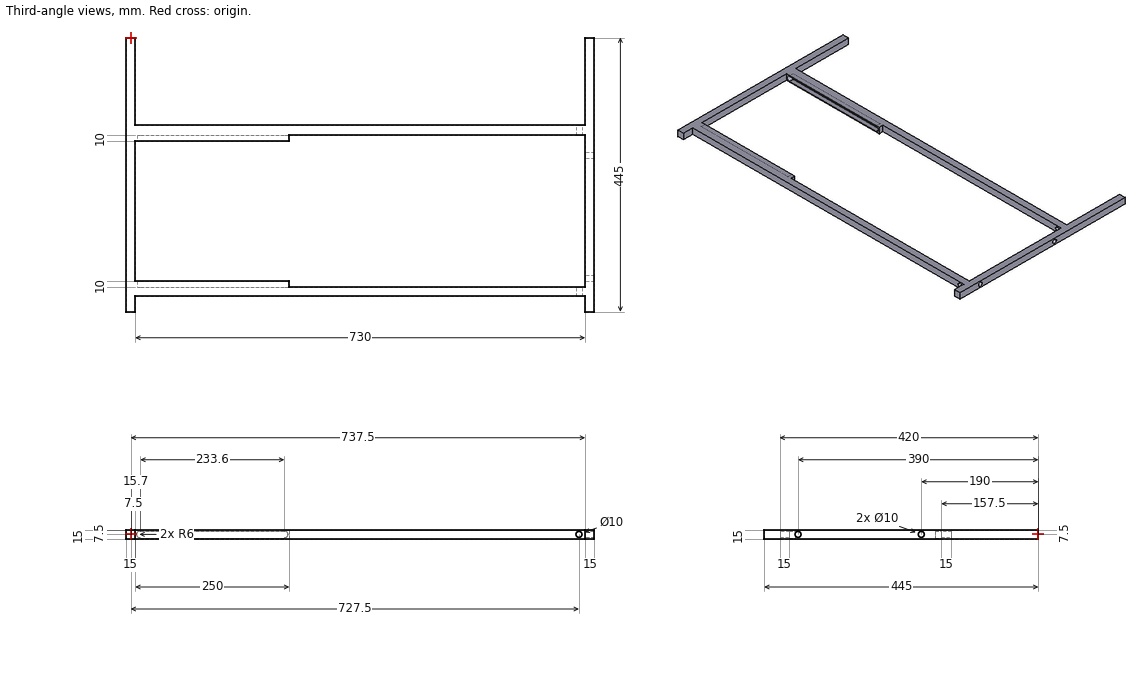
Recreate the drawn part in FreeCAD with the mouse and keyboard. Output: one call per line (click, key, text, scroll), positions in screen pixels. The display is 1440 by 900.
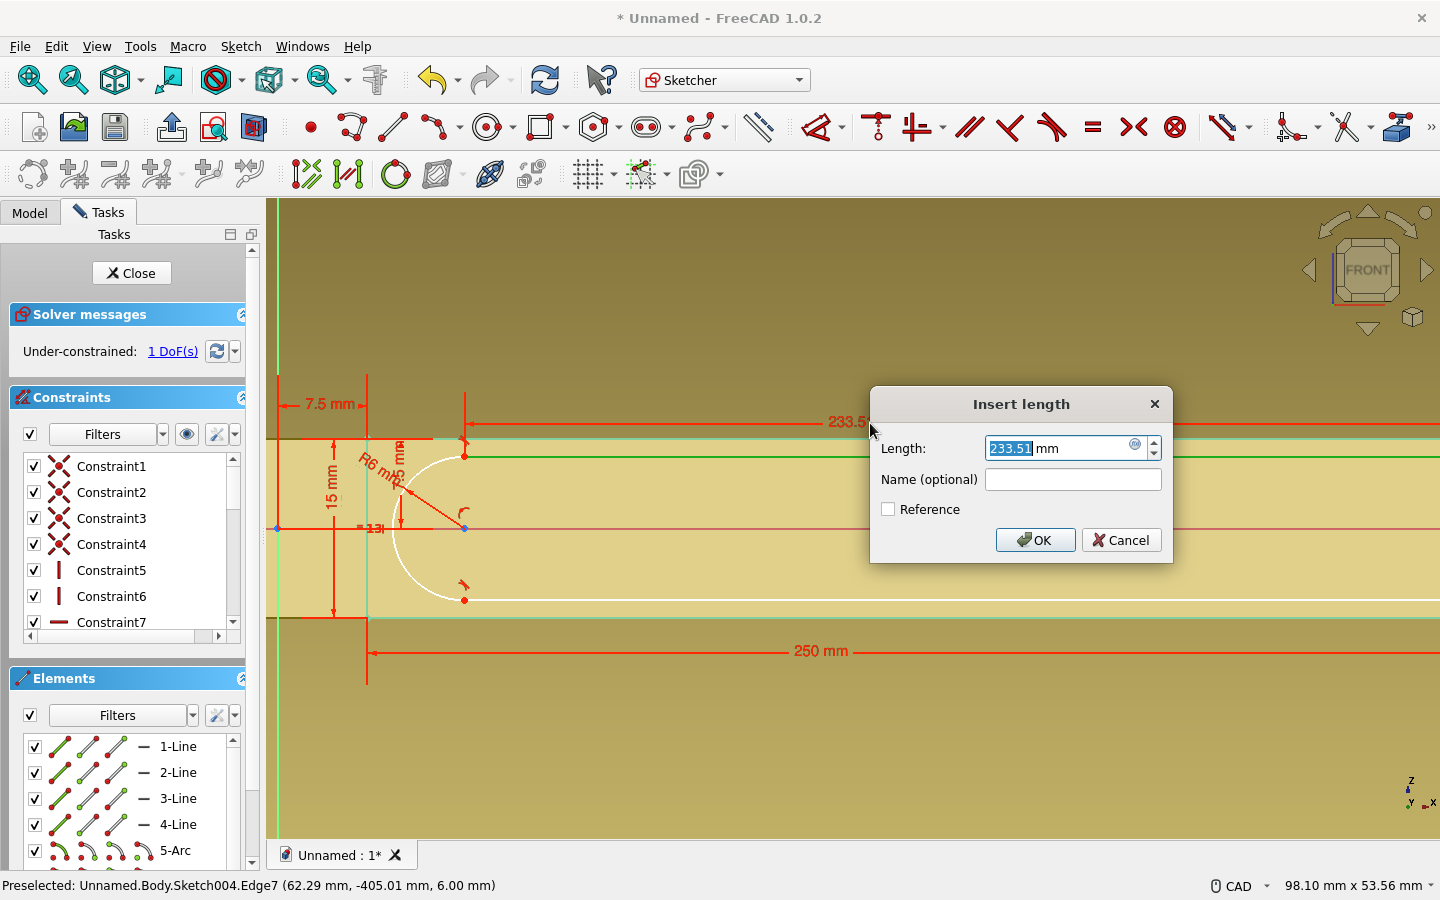
text(233.6)
key(Return)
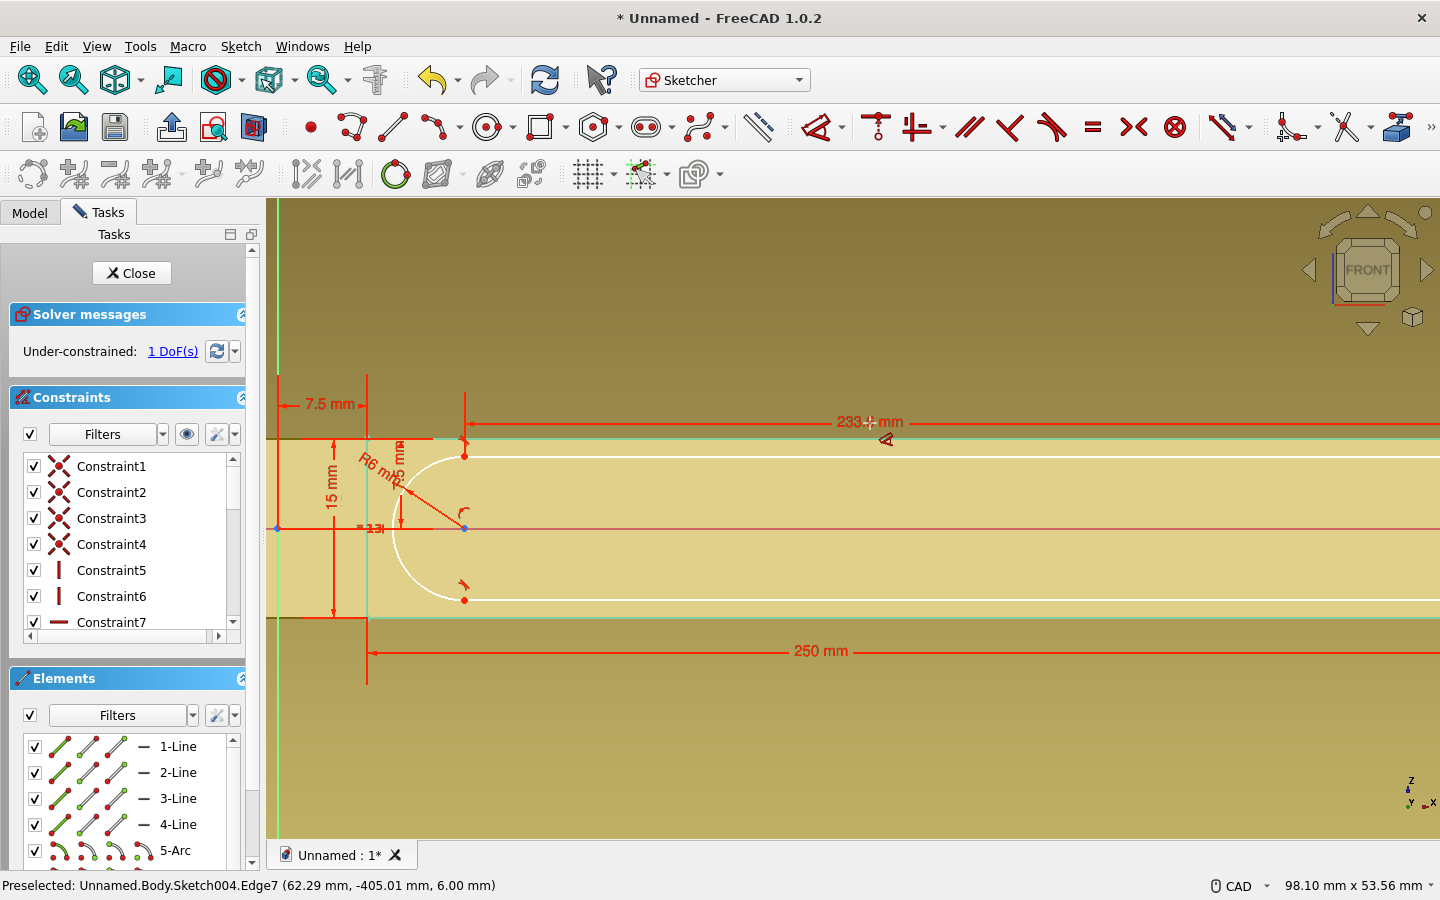
scroll(446, 515, down, 7)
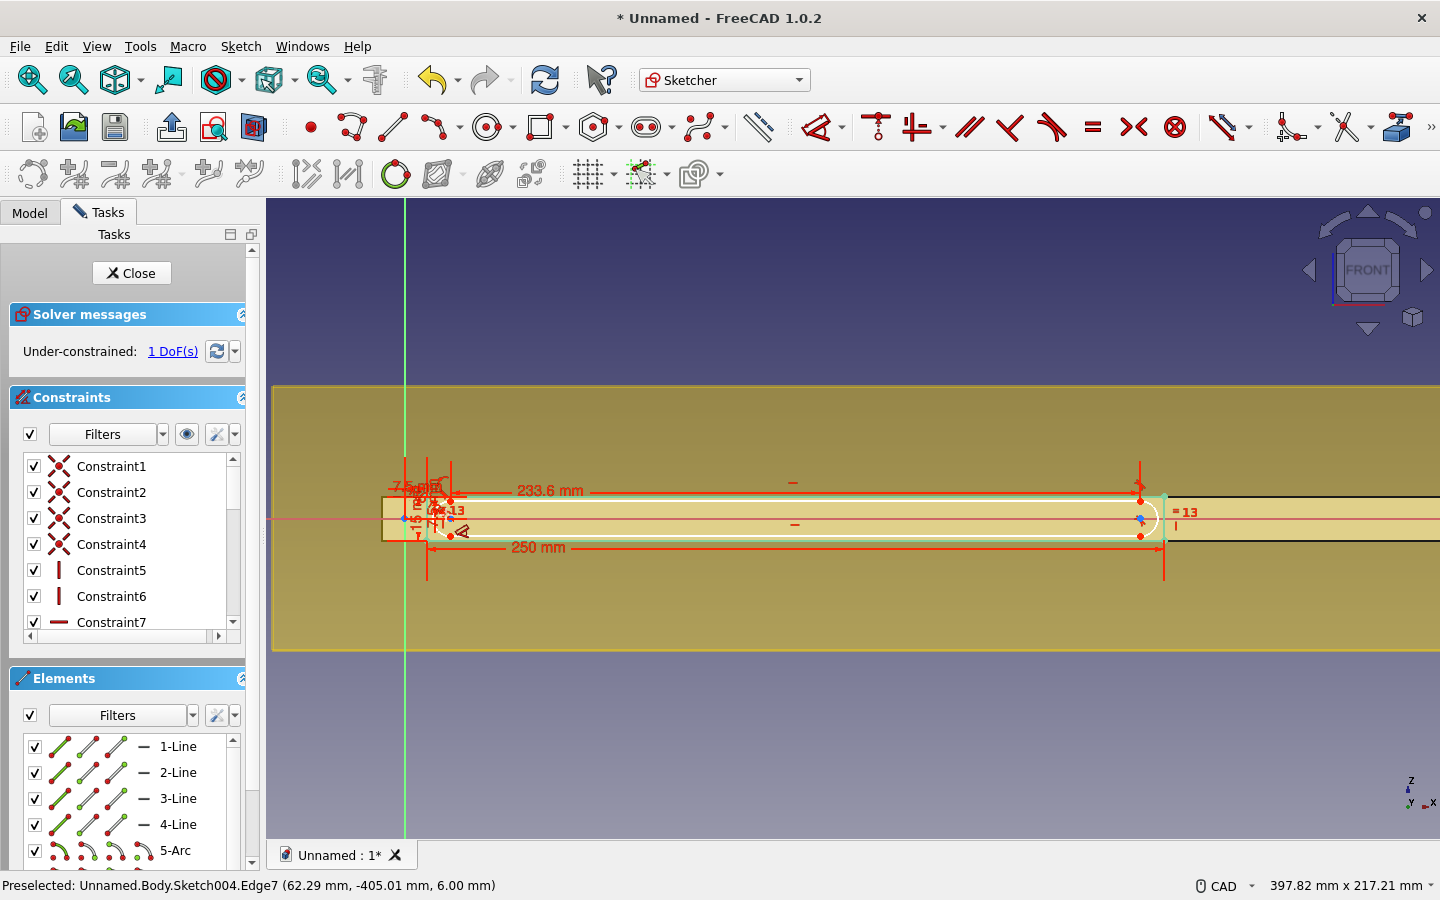
click(451, 501)
click(428, 467)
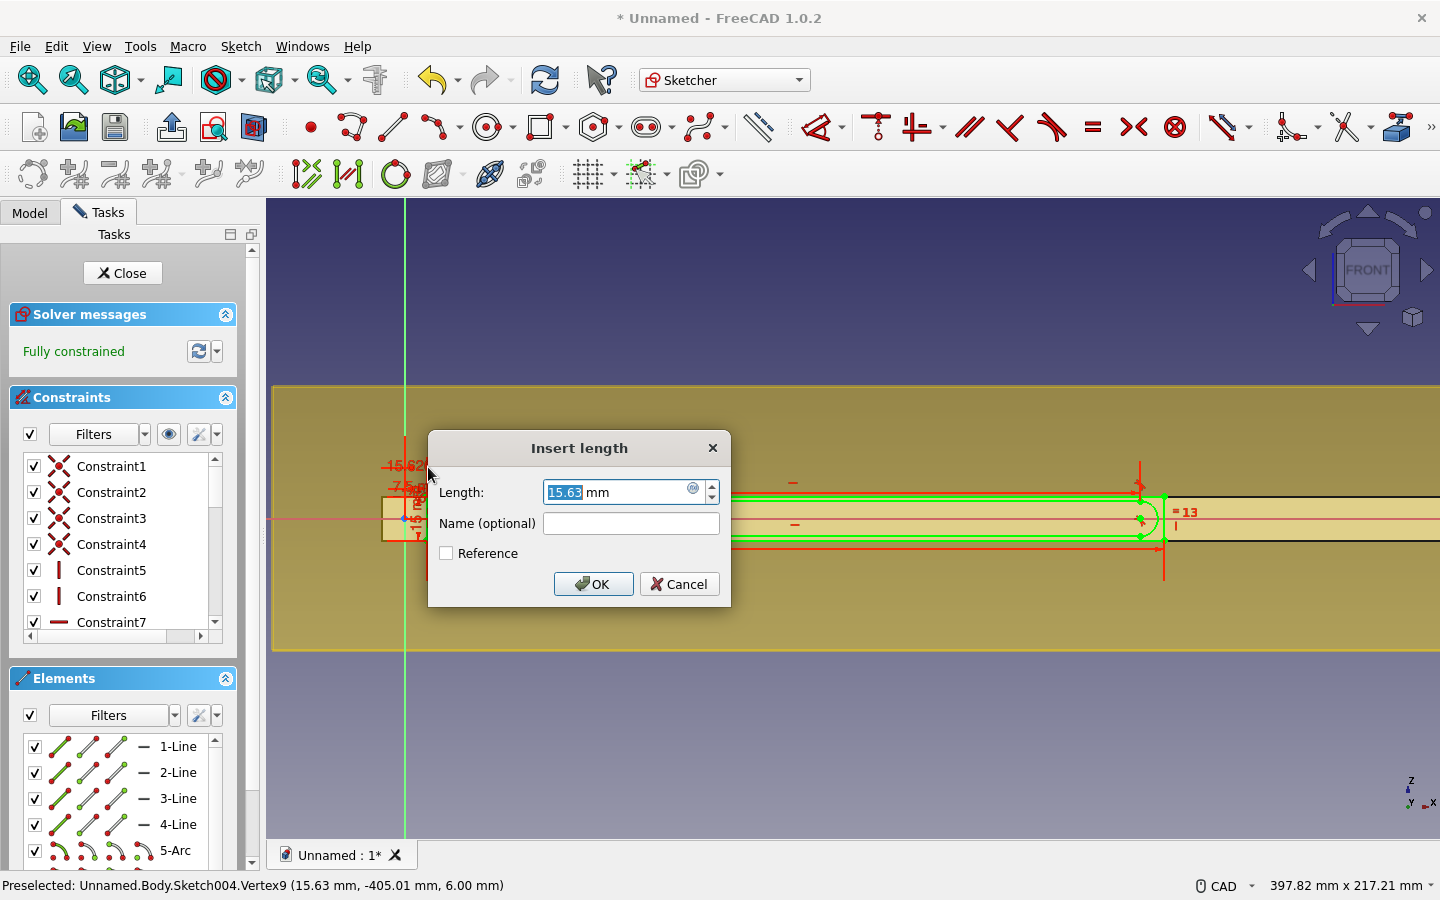
text(15.7)
key(Return)
key(Escape)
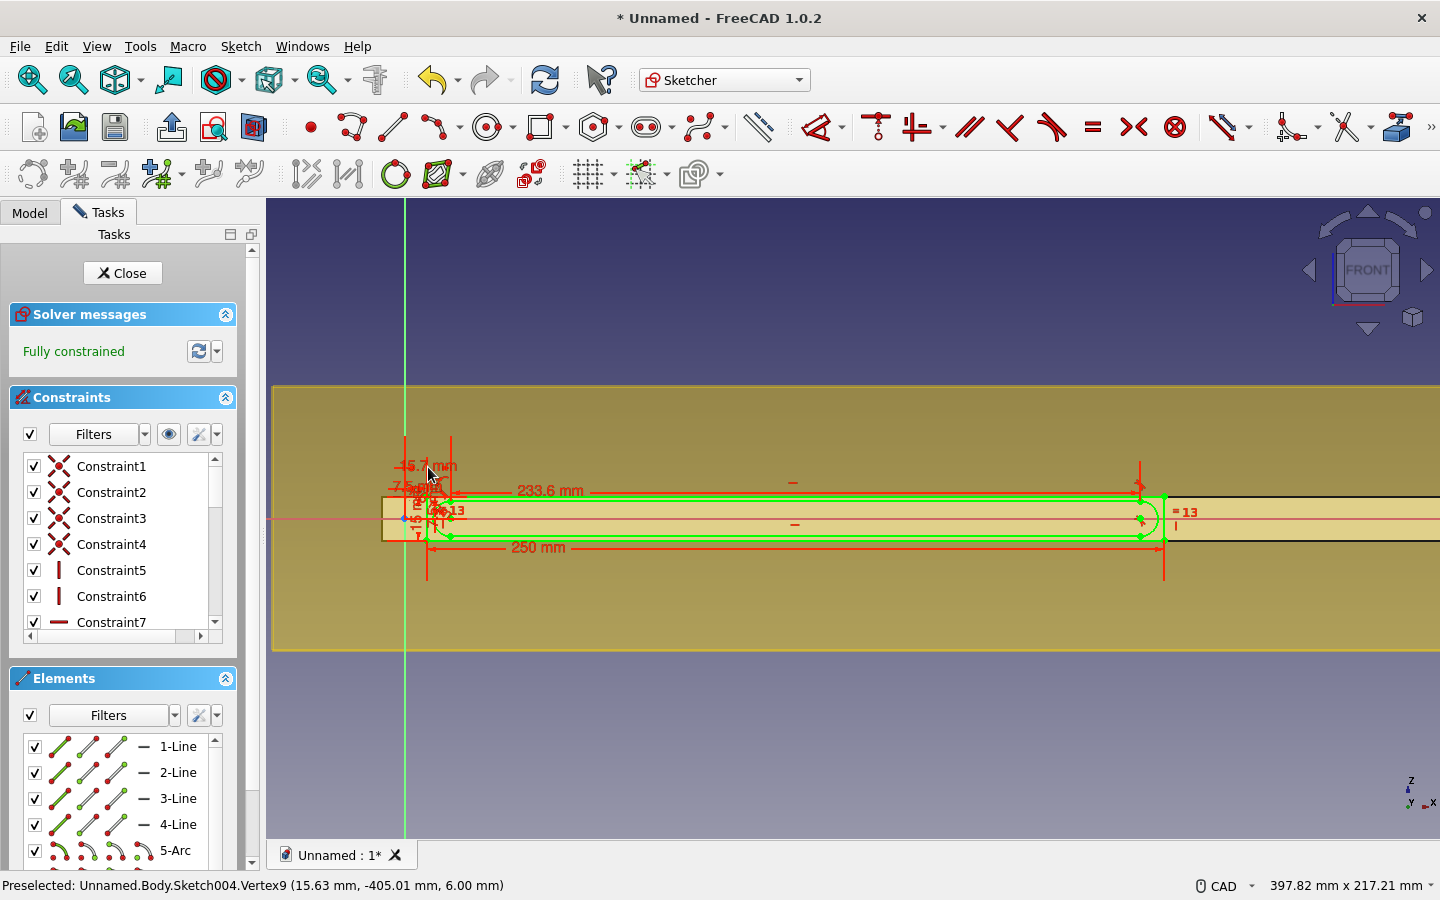
click(123, 273)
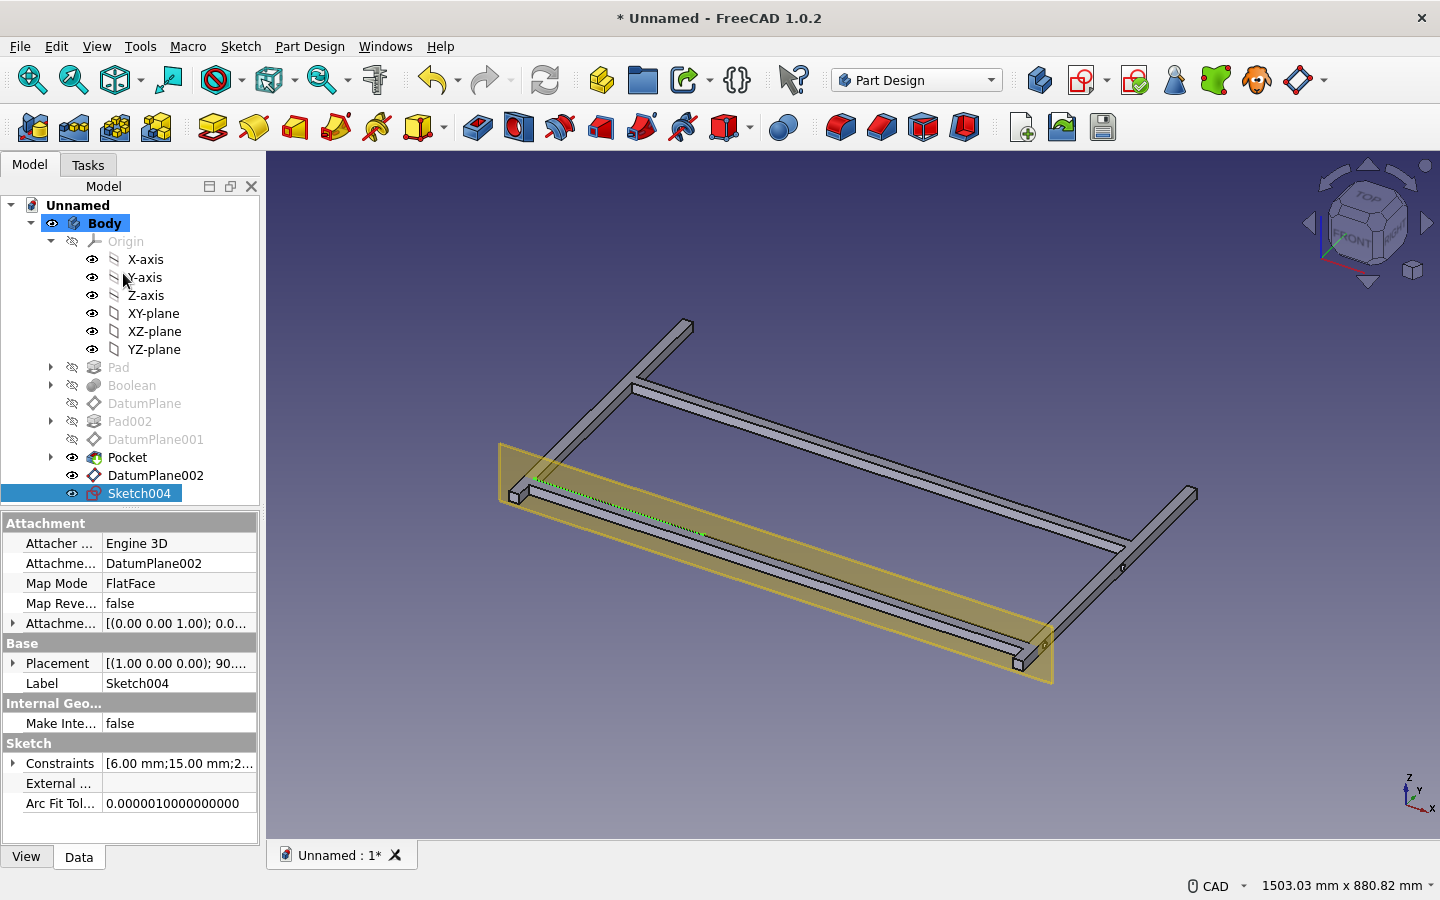
click(213, 128)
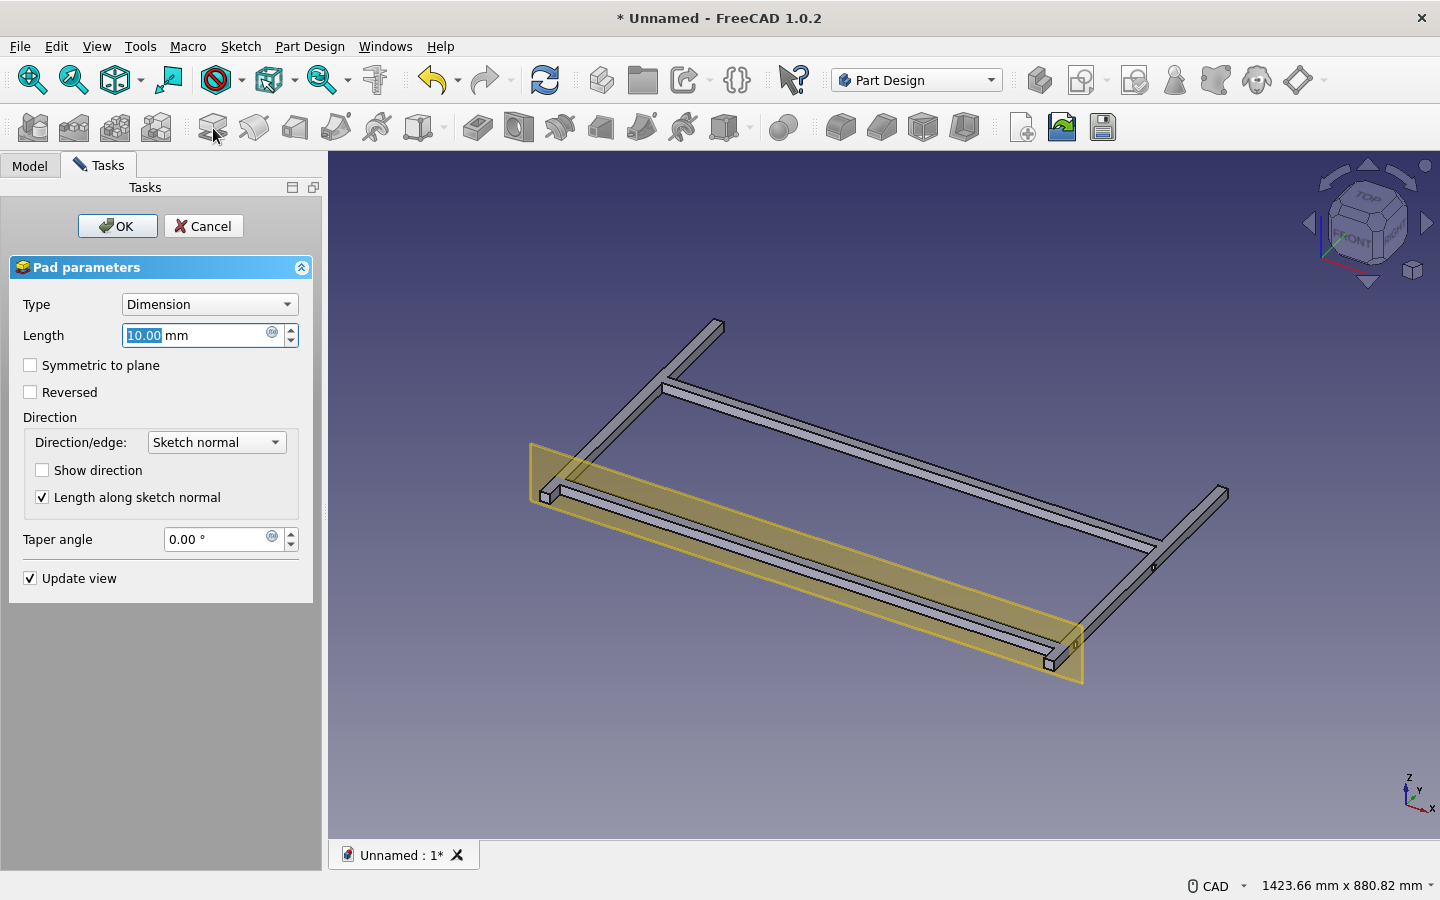
text(10)
key(Tab)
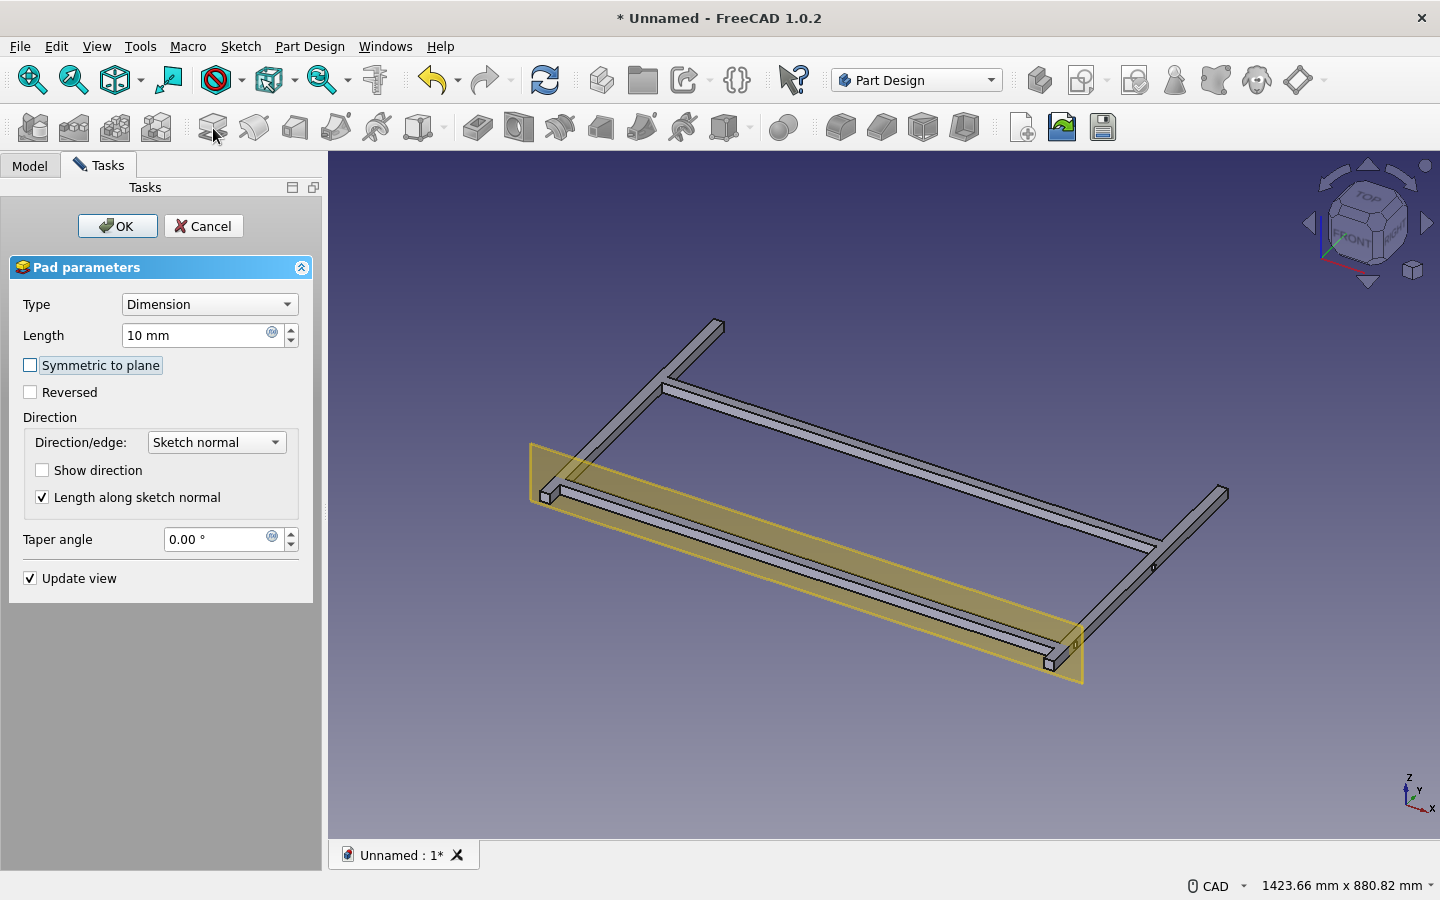
click(31, 392)